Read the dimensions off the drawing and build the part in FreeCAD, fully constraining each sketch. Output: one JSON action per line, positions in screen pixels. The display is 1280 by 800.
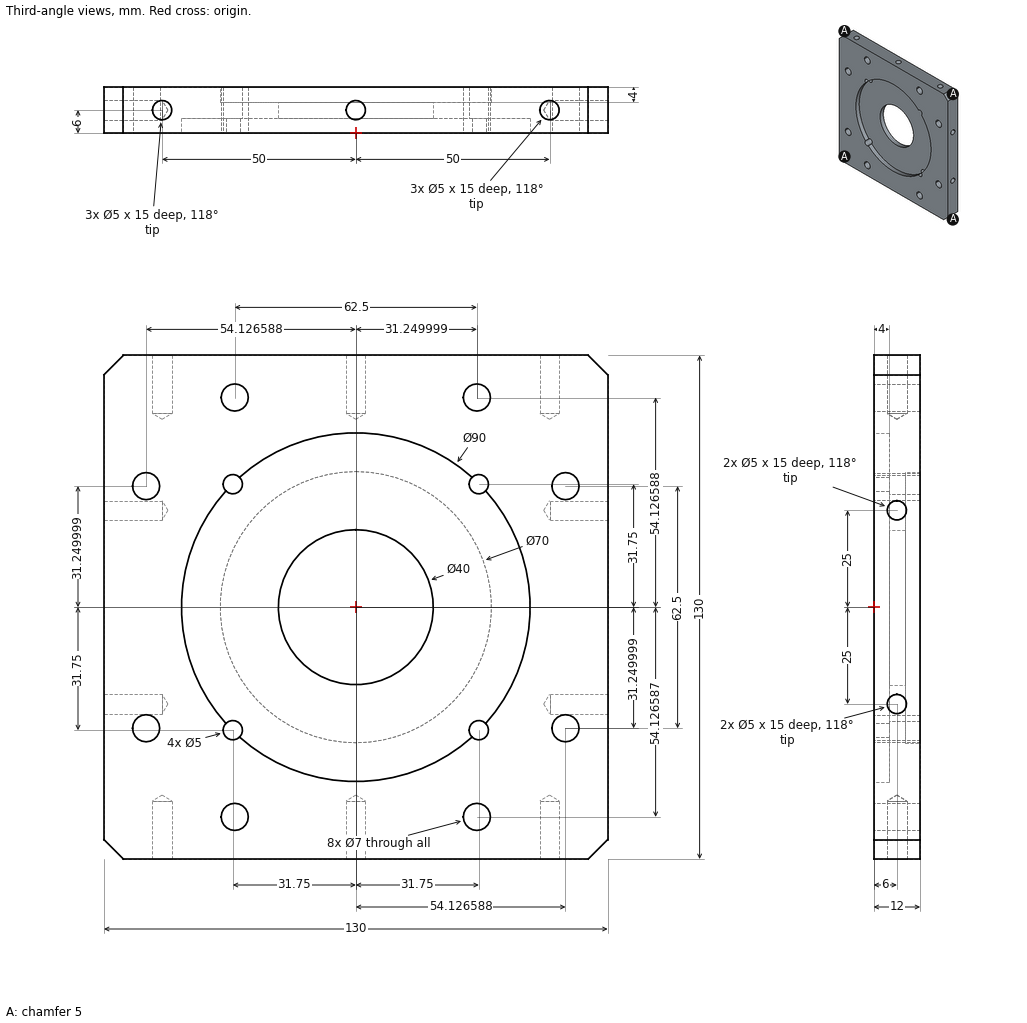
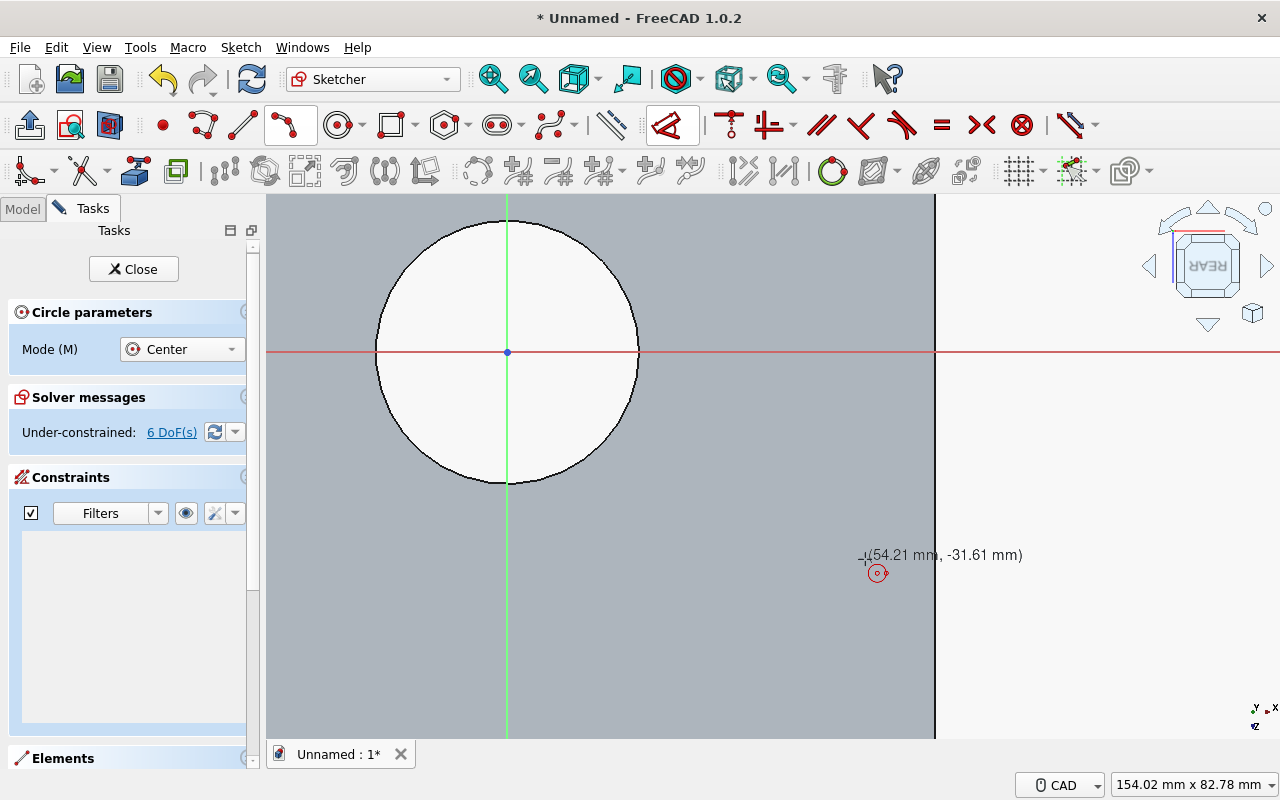
{"action": "left_click", "coordinate": [864, 558]}
{"action": "left_click", "coordinate": [880, 542]}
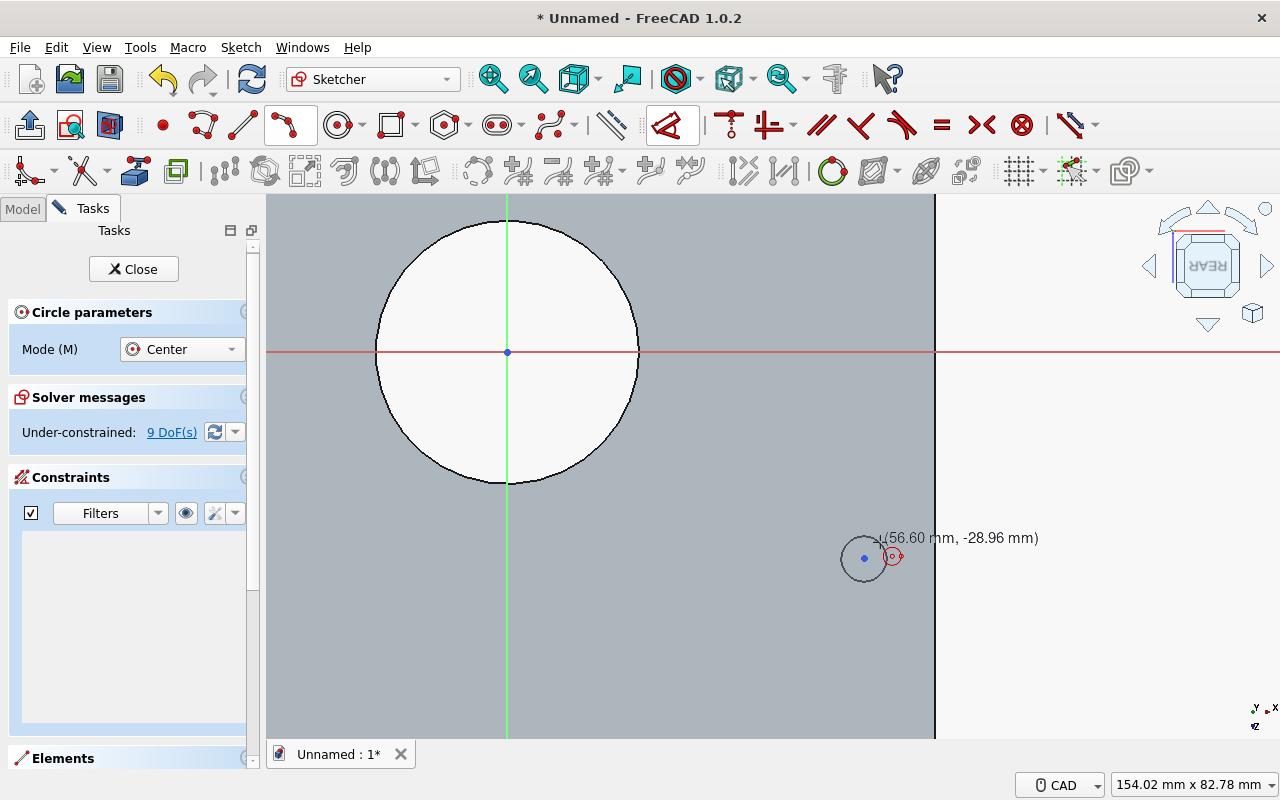
{"action": "left_click", "coordinate": [713, 709]}
{"action": "left_click", "coordinate": [729, 692]}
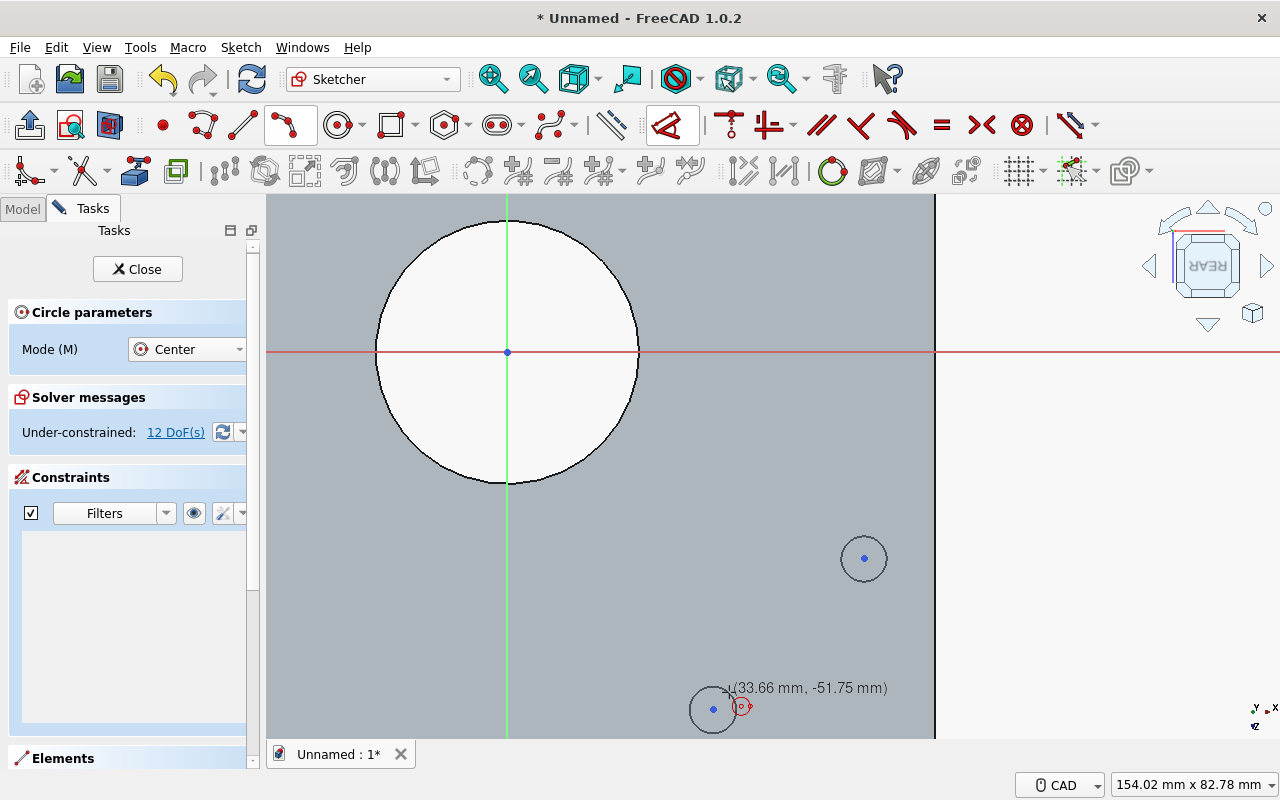
{"action": "left_click", "coordinate": [302, 709]}
{"action": "left_click", "coordinate": [318, 692]}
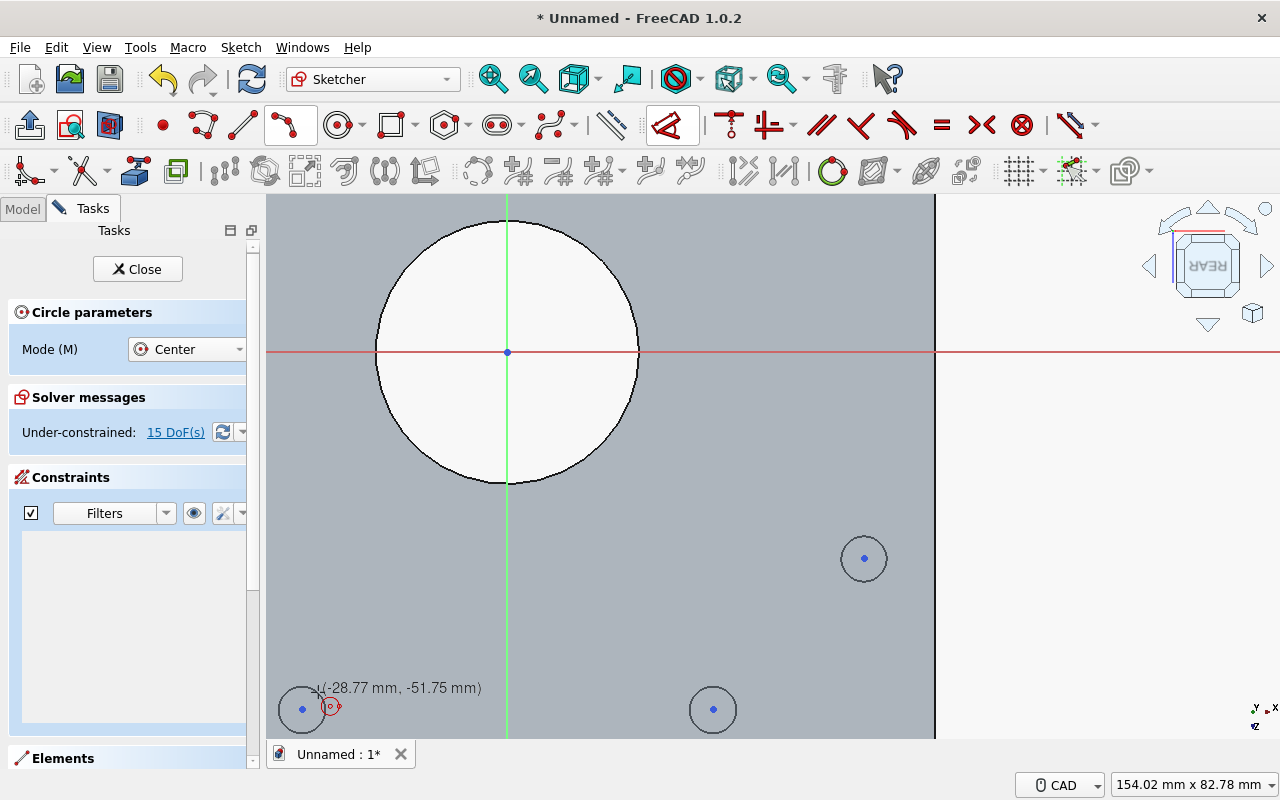
{"action": "scroll", "coordinate": [865, 560], "scroll_direction": "down", "scroll_amount": 4}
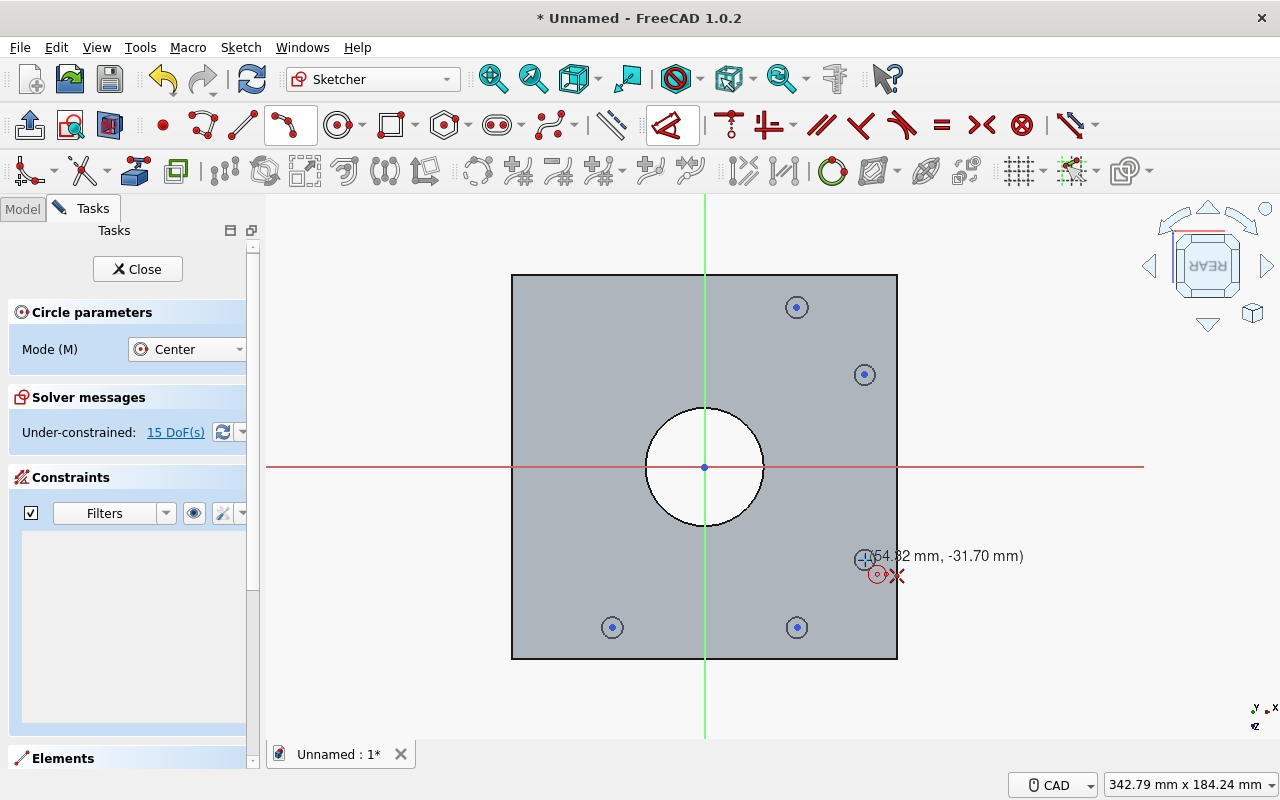
{"action": "scroll", "coordinate": [545, 559], "scroll_direction": "up", "scroll_amount": 4}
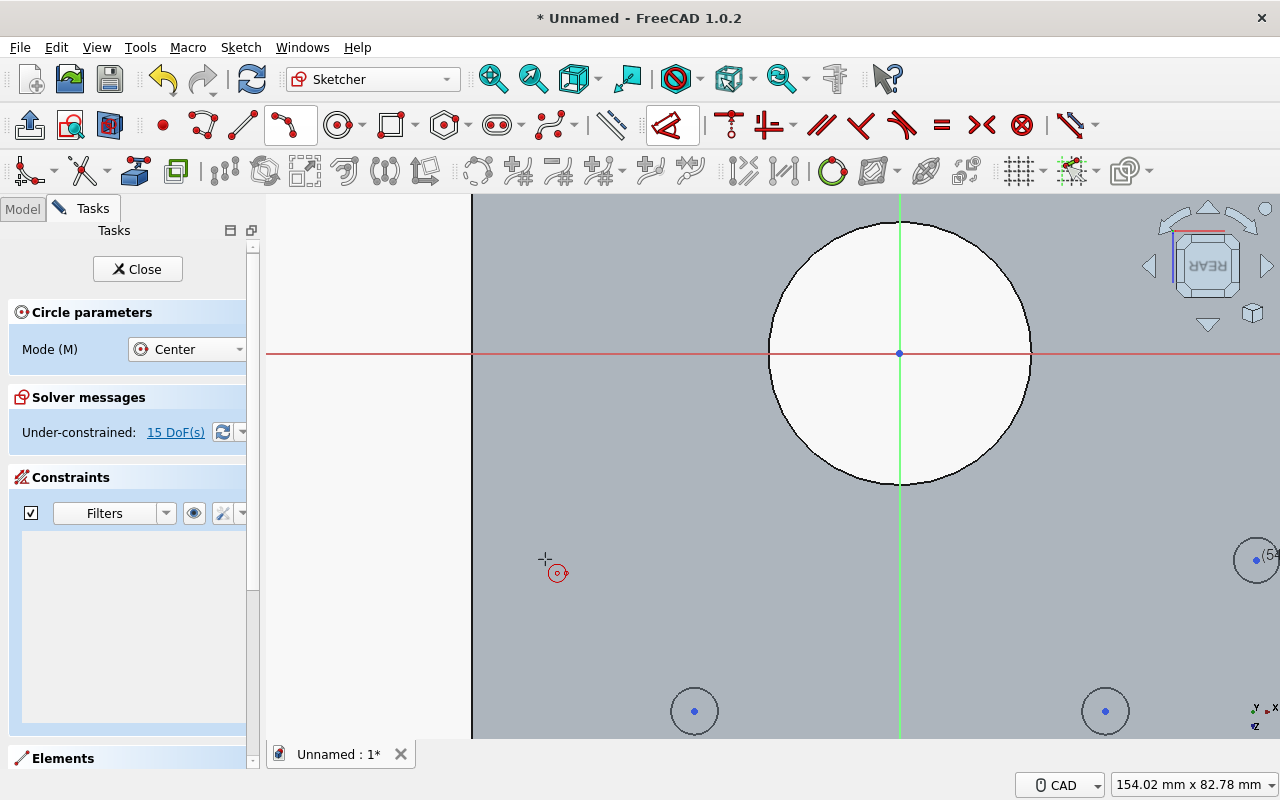
{"action": "left_click", "coordinate": [544, 559]}
{"action": "left_click", "coordinate": [560, 543]}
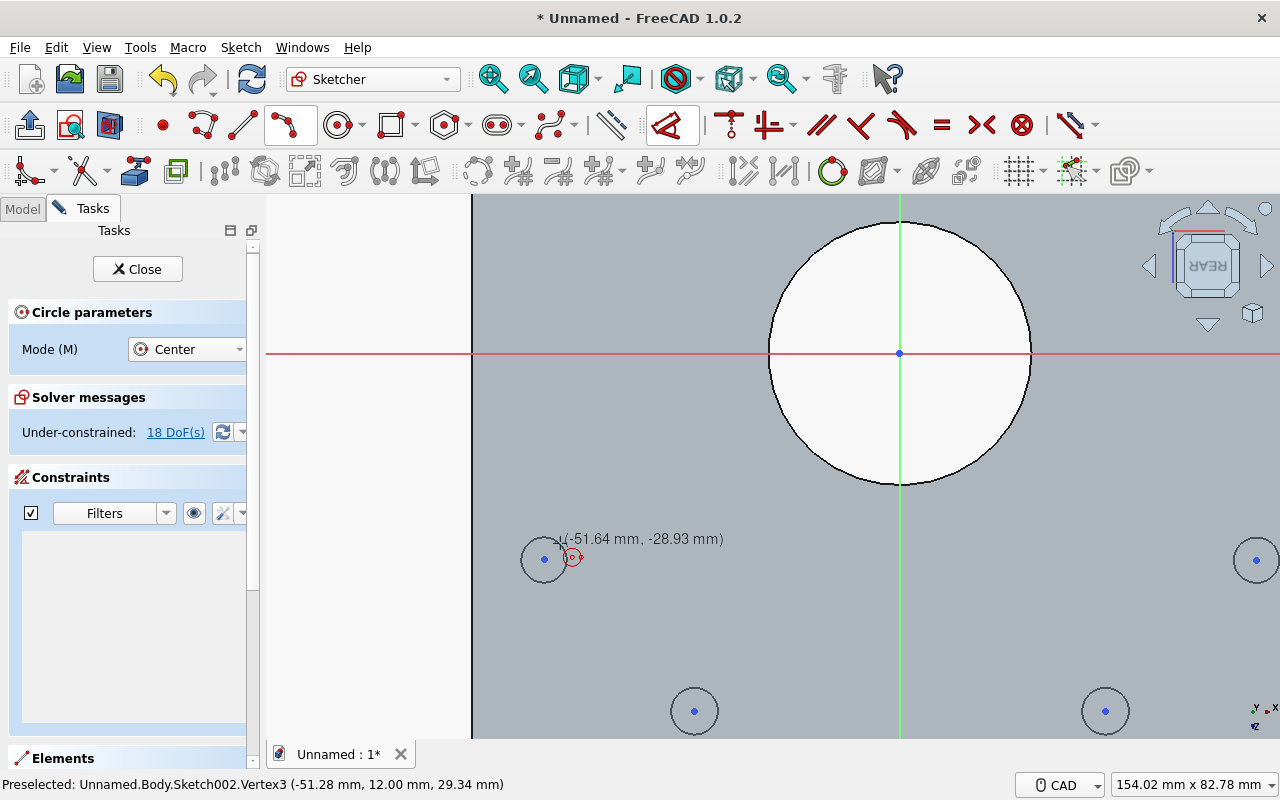
{"action": "scroll", "coordinate": [545, 559], "scroll_direction": "down", "scroll_amount": 4}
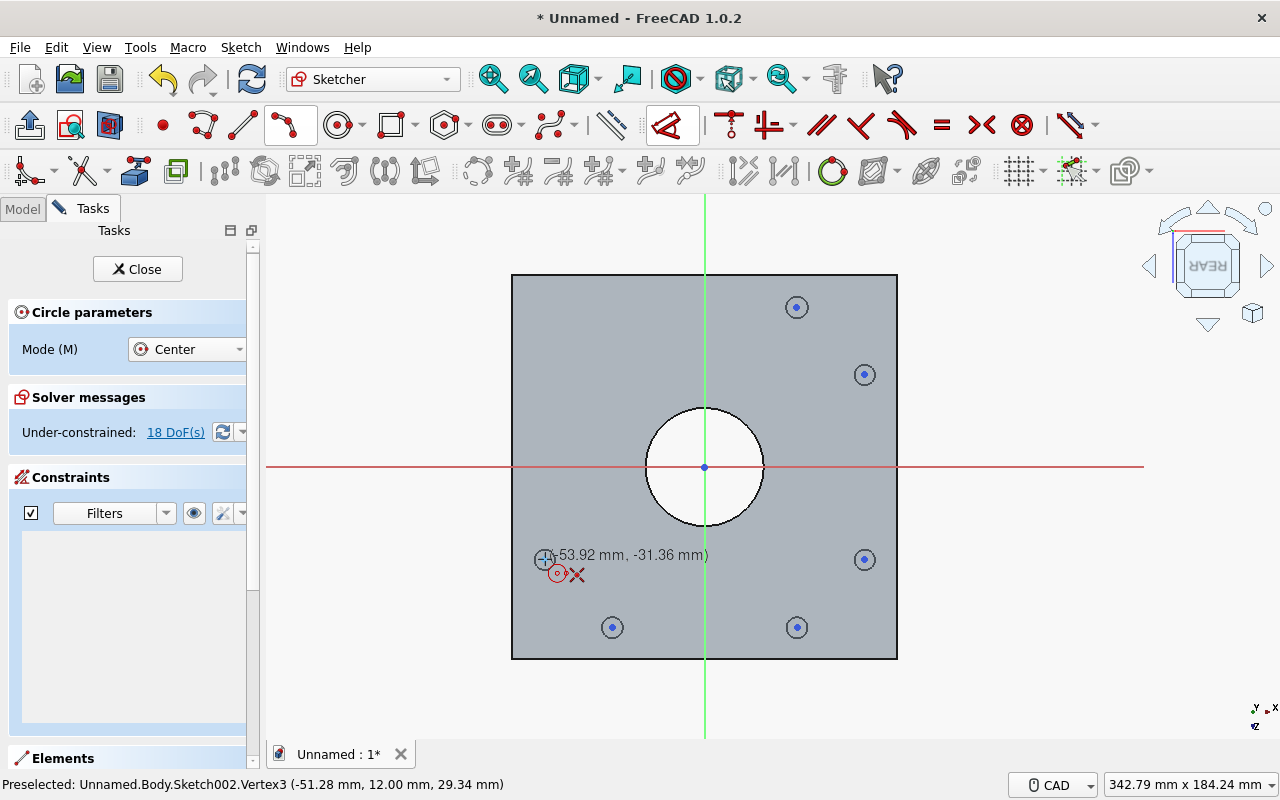
{"action": "scroll", "coordinate": [545, 375], "scroll_direction": "up", "scroll_amount": 4}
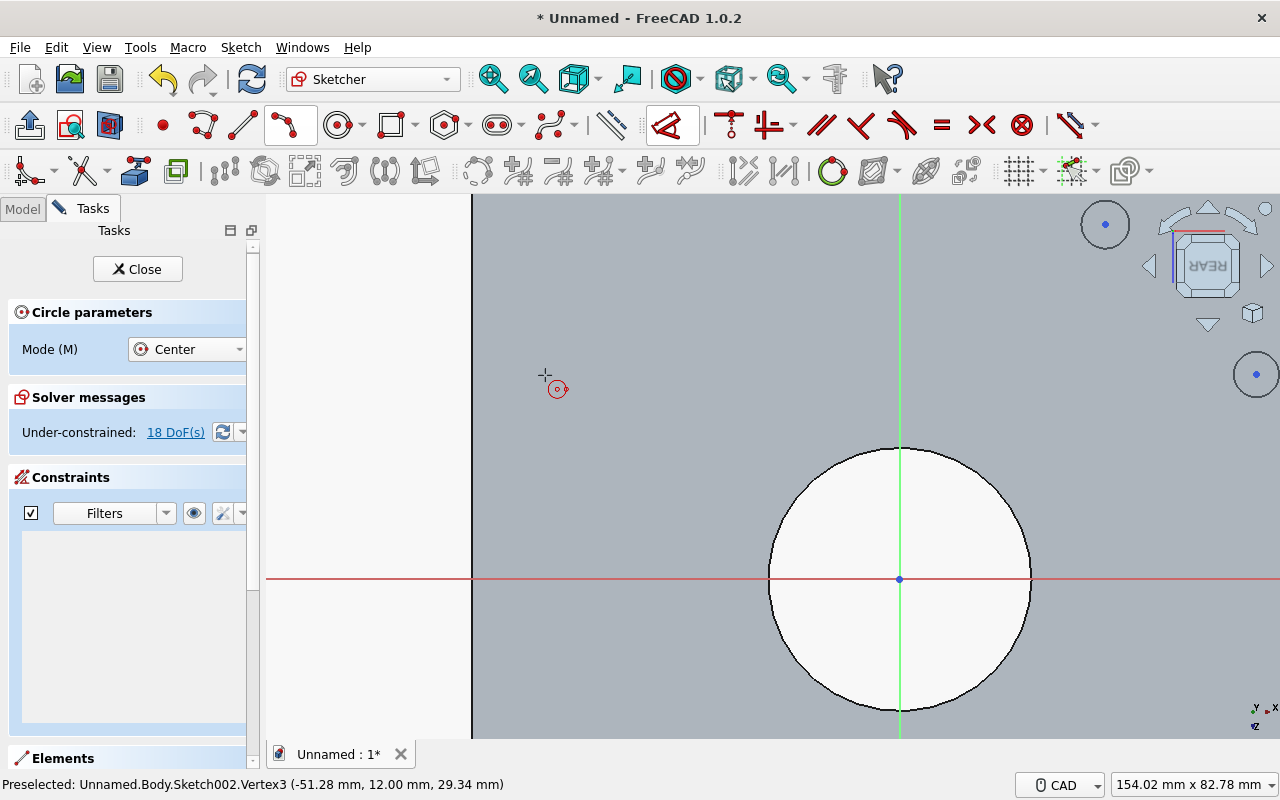
{"action": "left_click", "coordinate": [544, 374]}
{"action": "left_click", "coordinate": [560, 357]}